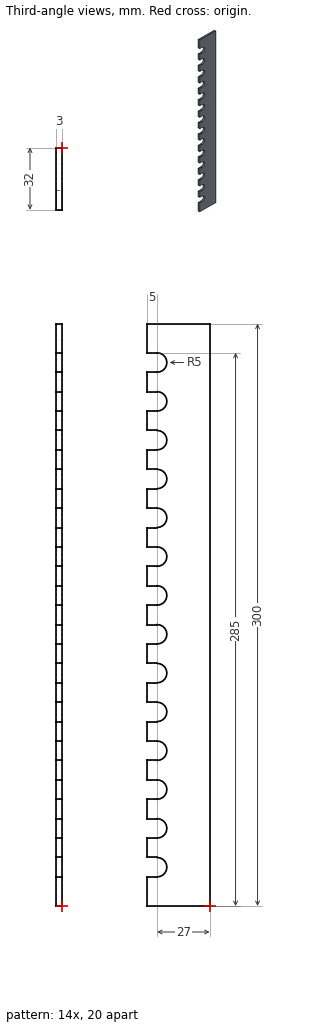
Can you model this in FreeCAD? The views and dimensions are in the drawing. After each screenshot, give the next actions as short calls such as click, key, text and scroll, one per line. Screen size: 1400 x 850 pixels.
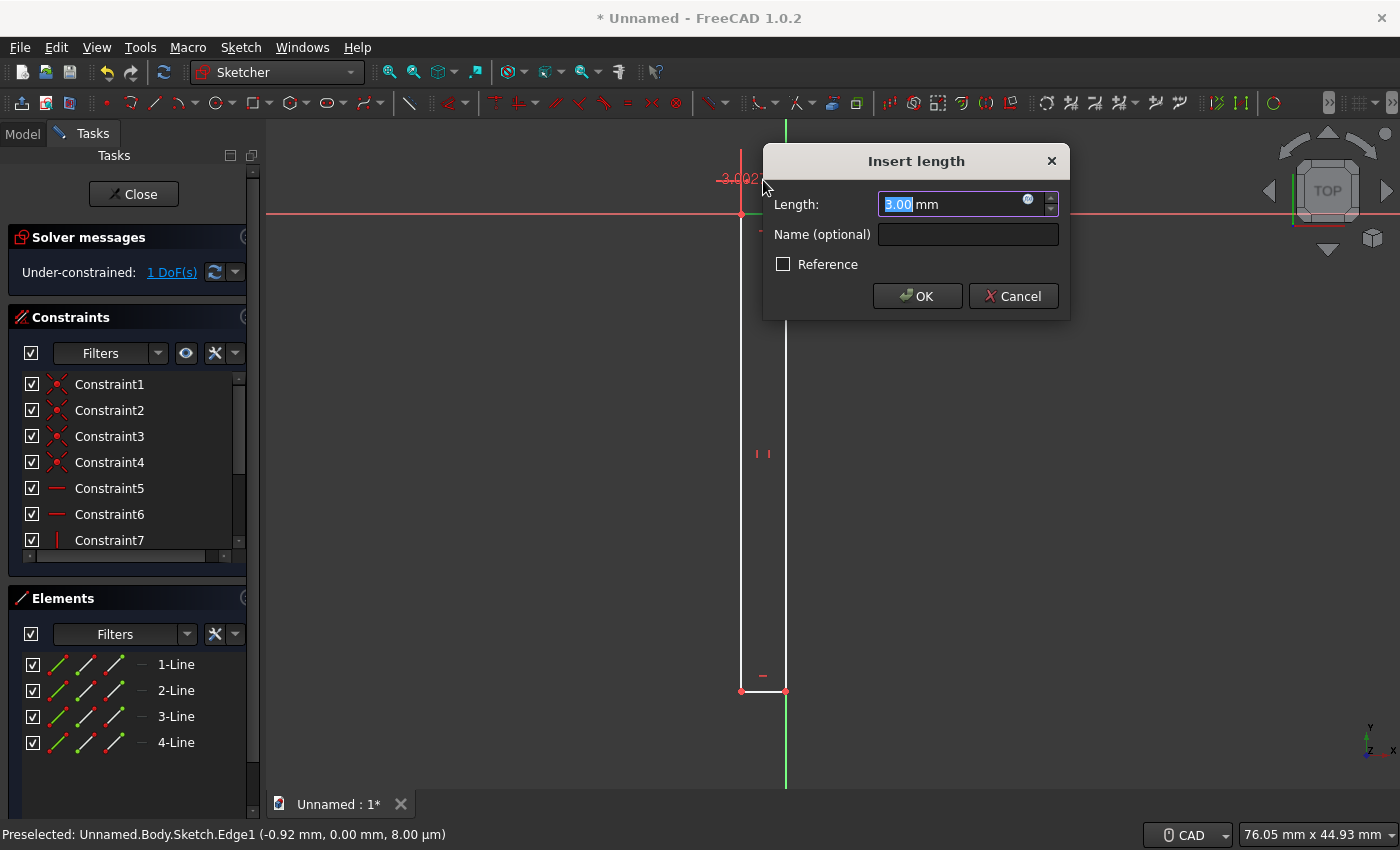
text(3)
key(Return)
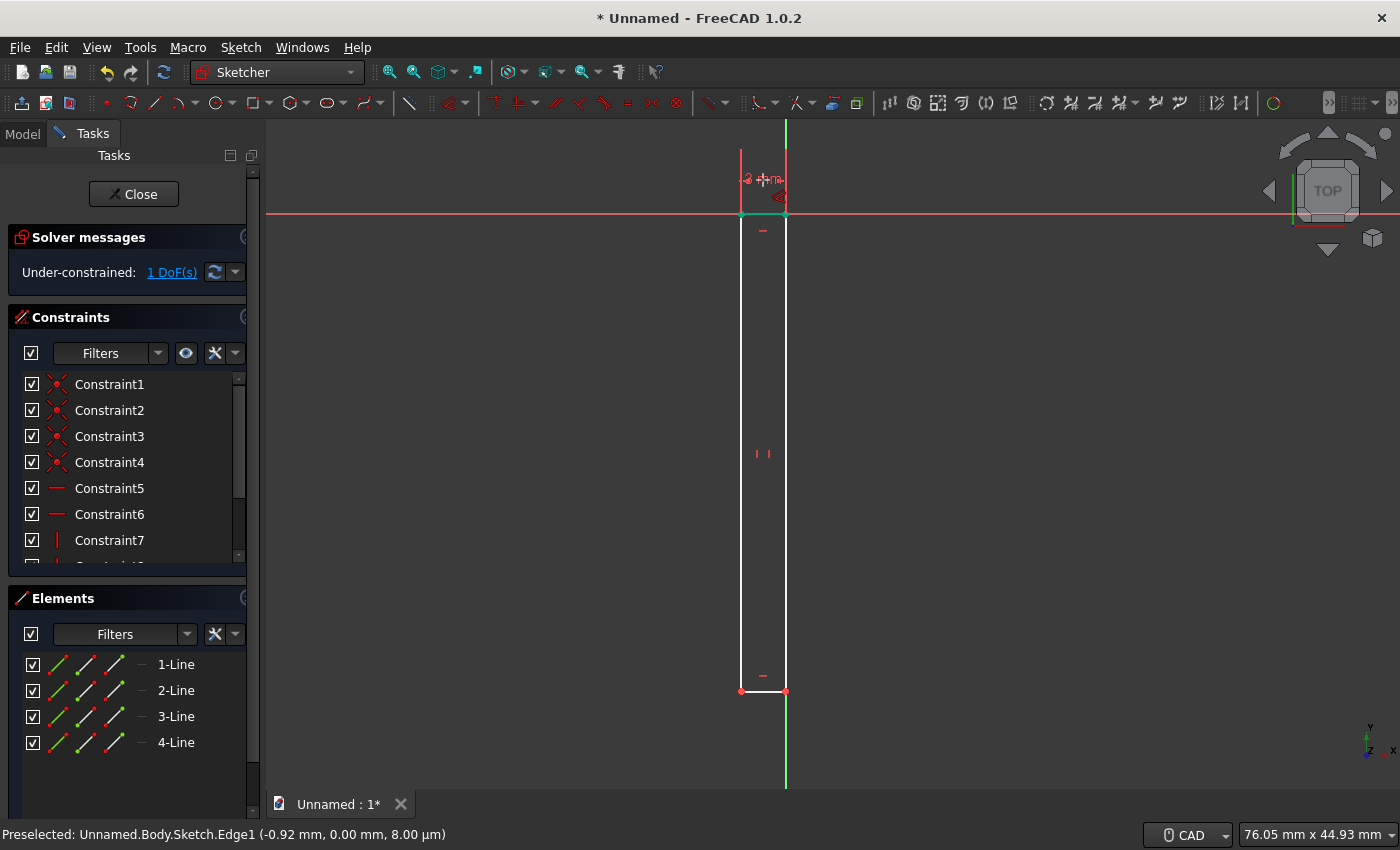
click(741, 357)
click(707, 453)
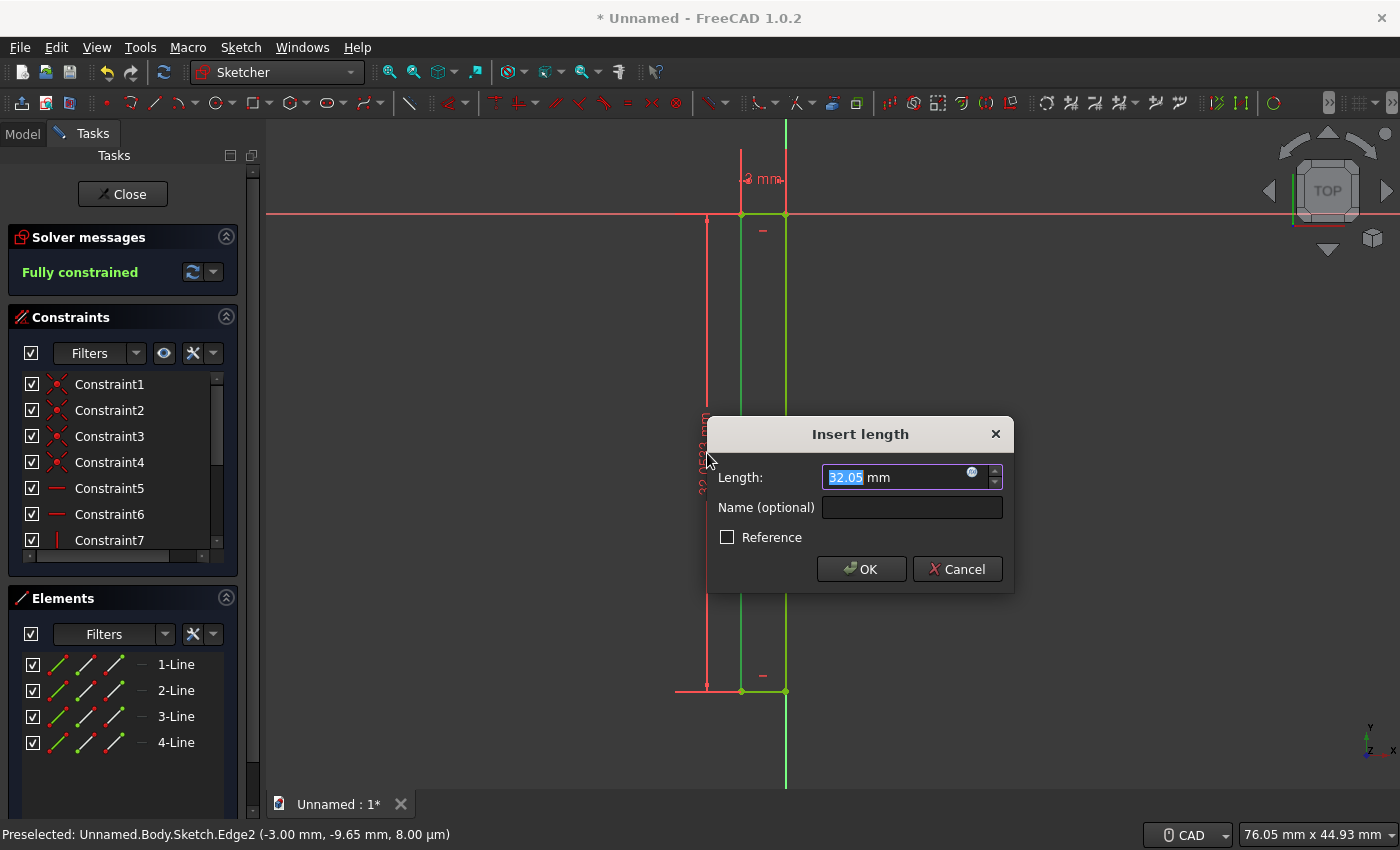
text(32)
key(Return)
key(Escape)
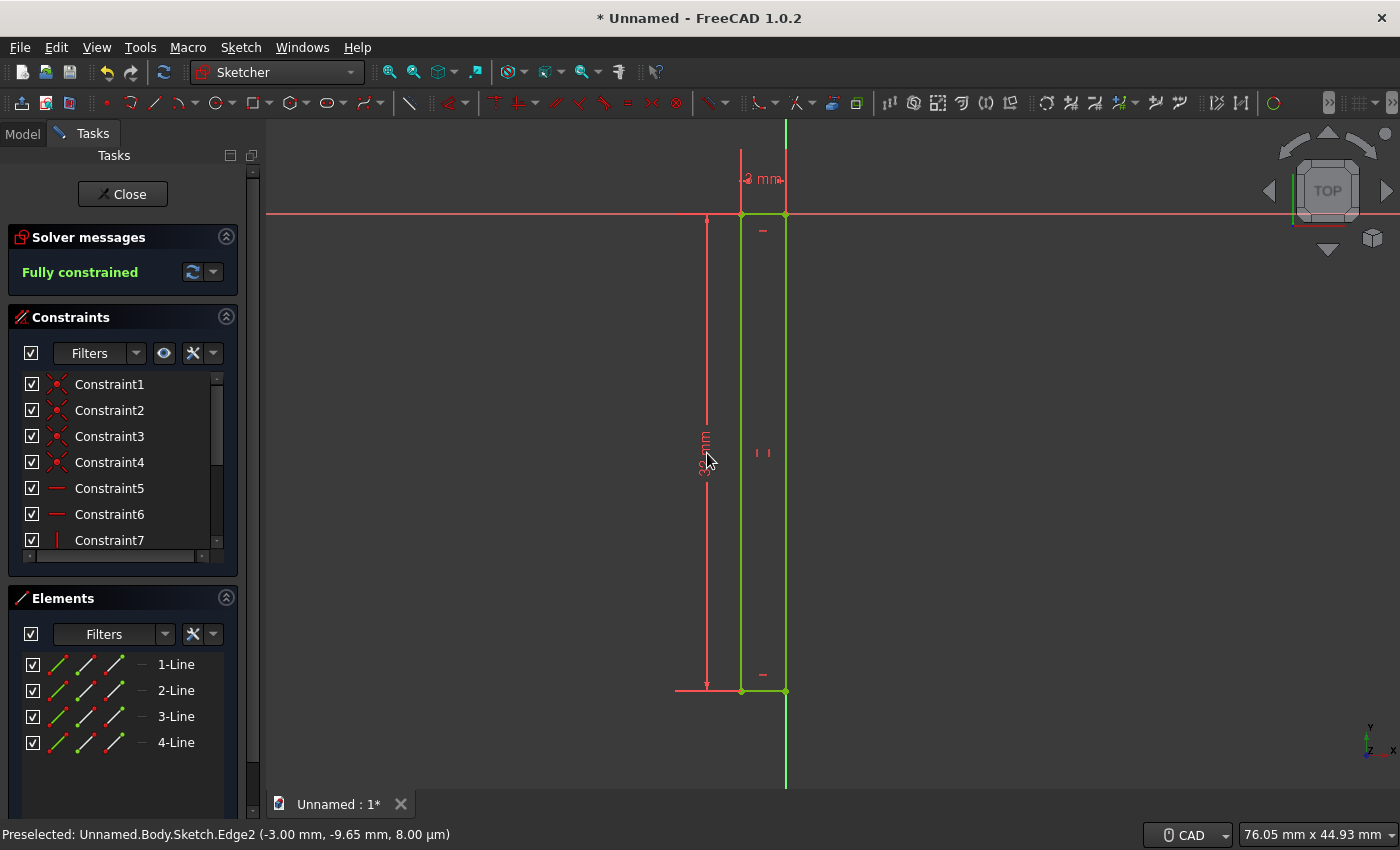
click(123, 194)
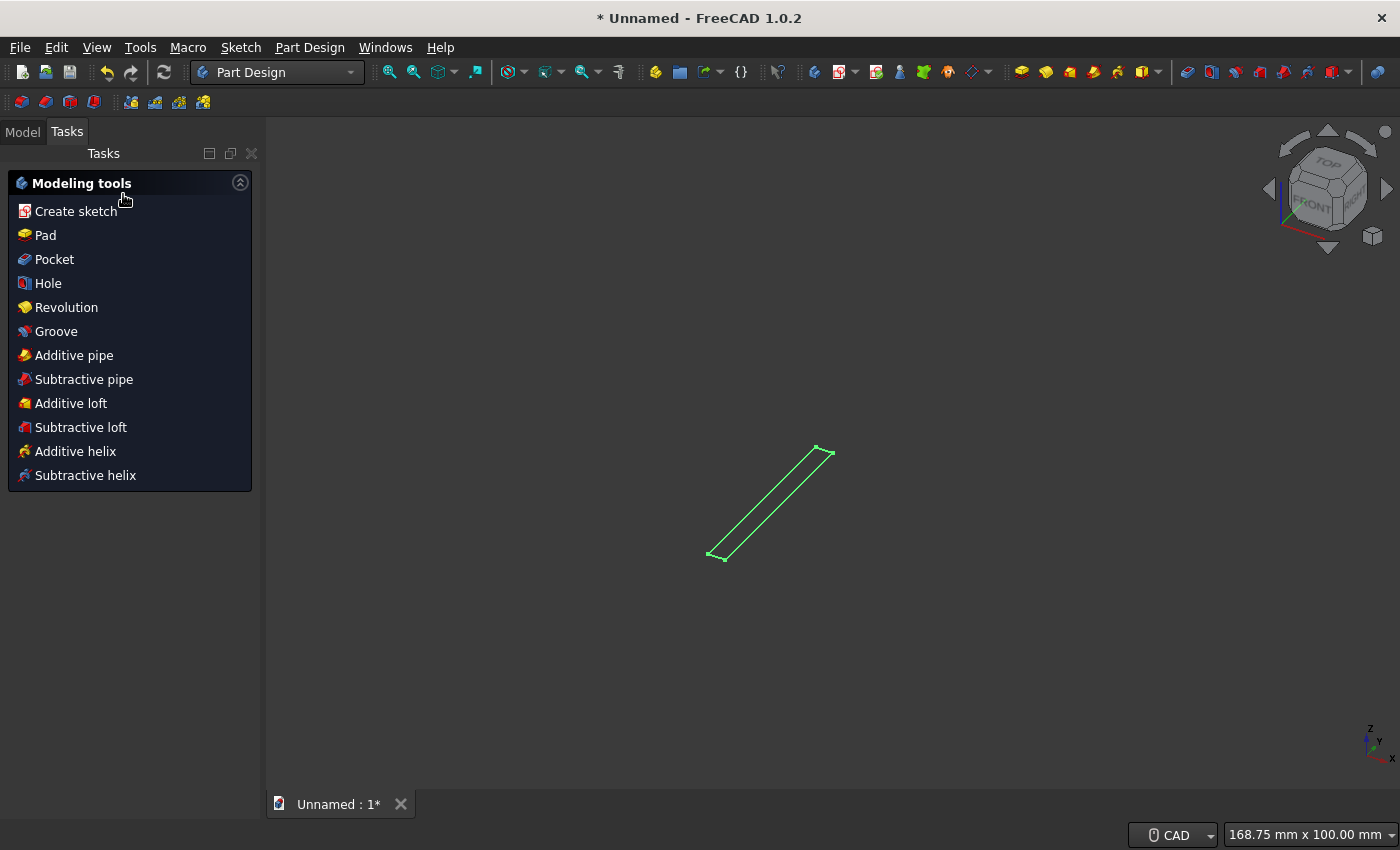
click(1022, 72)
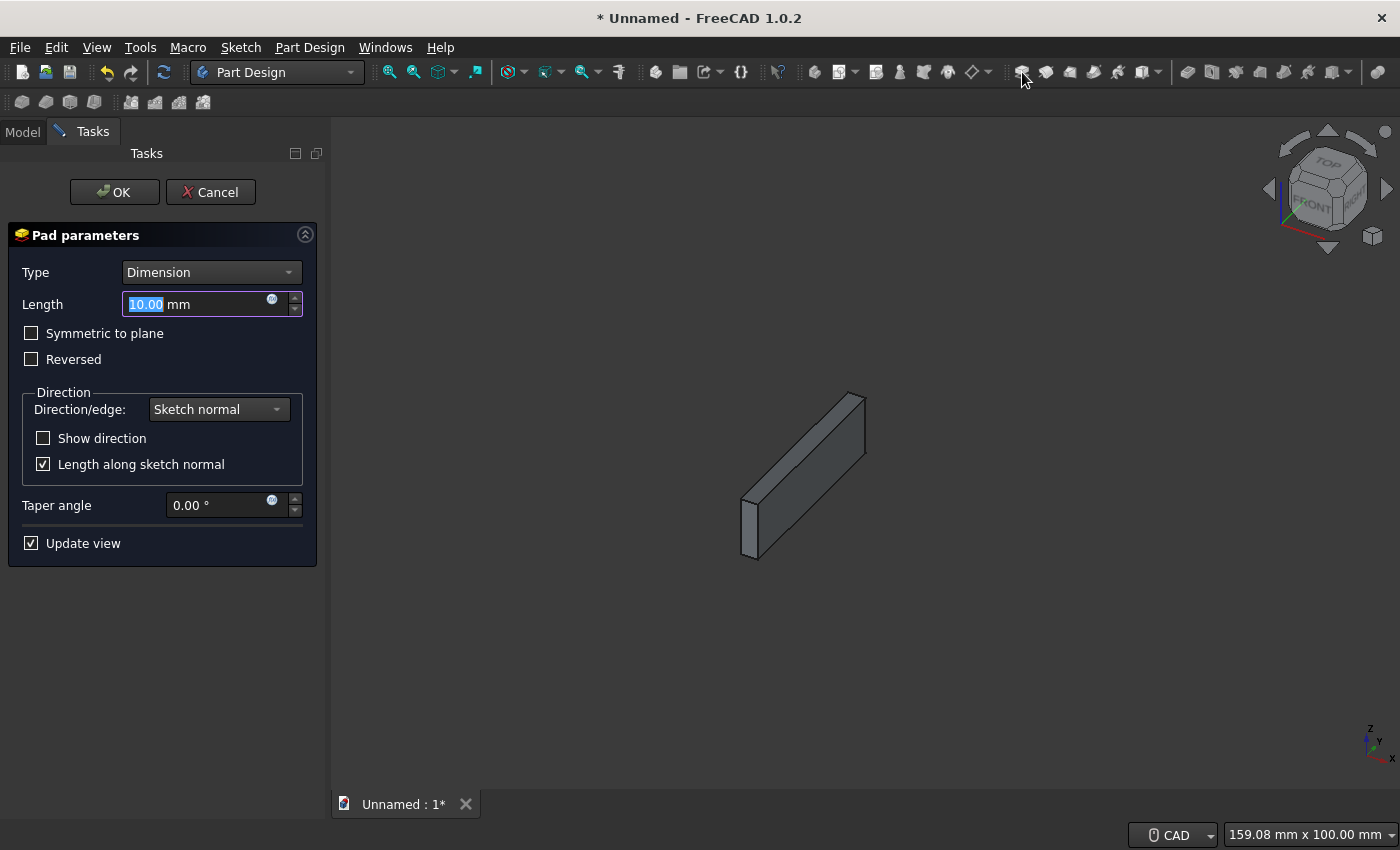
text(300)
key(Tab)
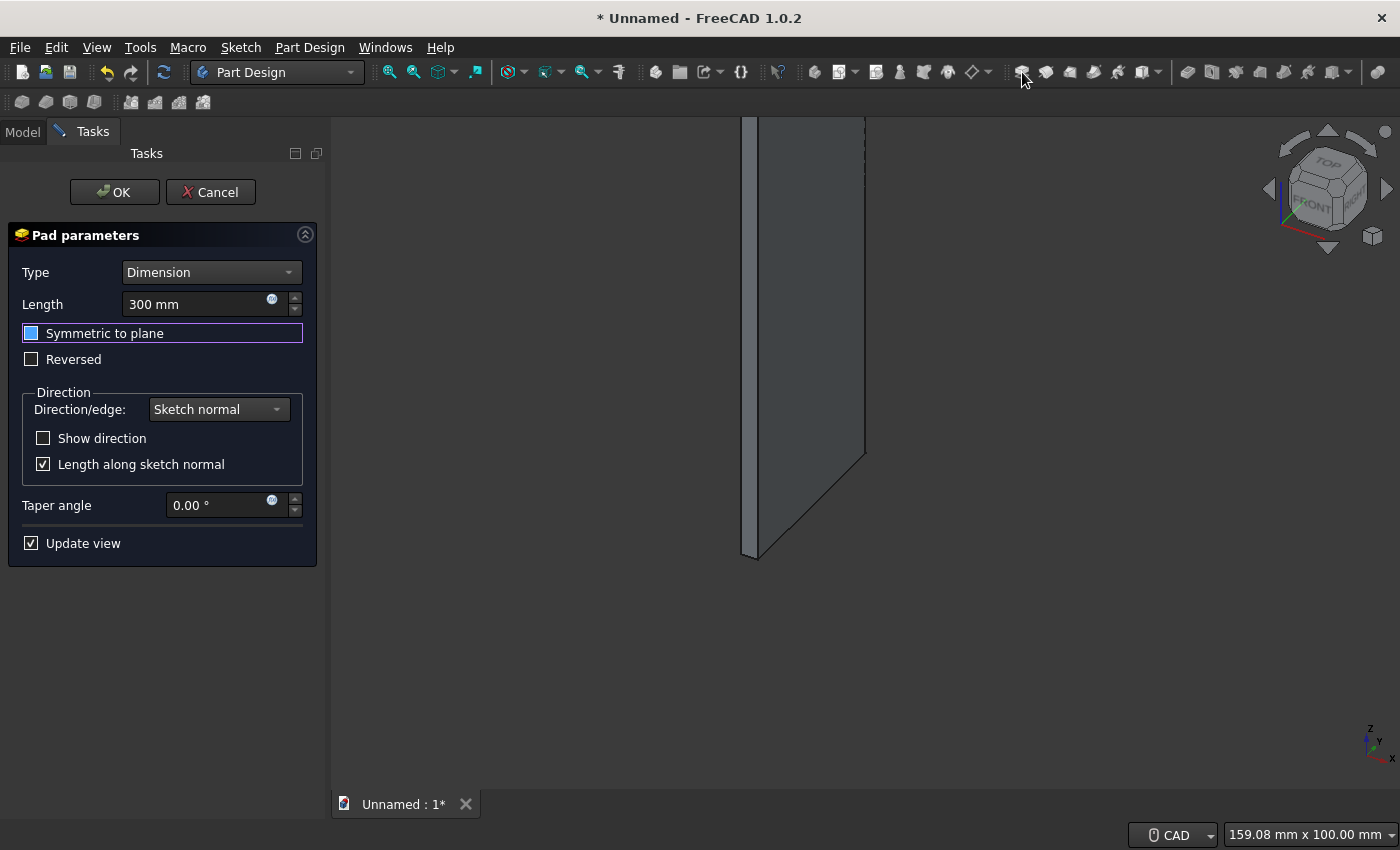
click(115, 192)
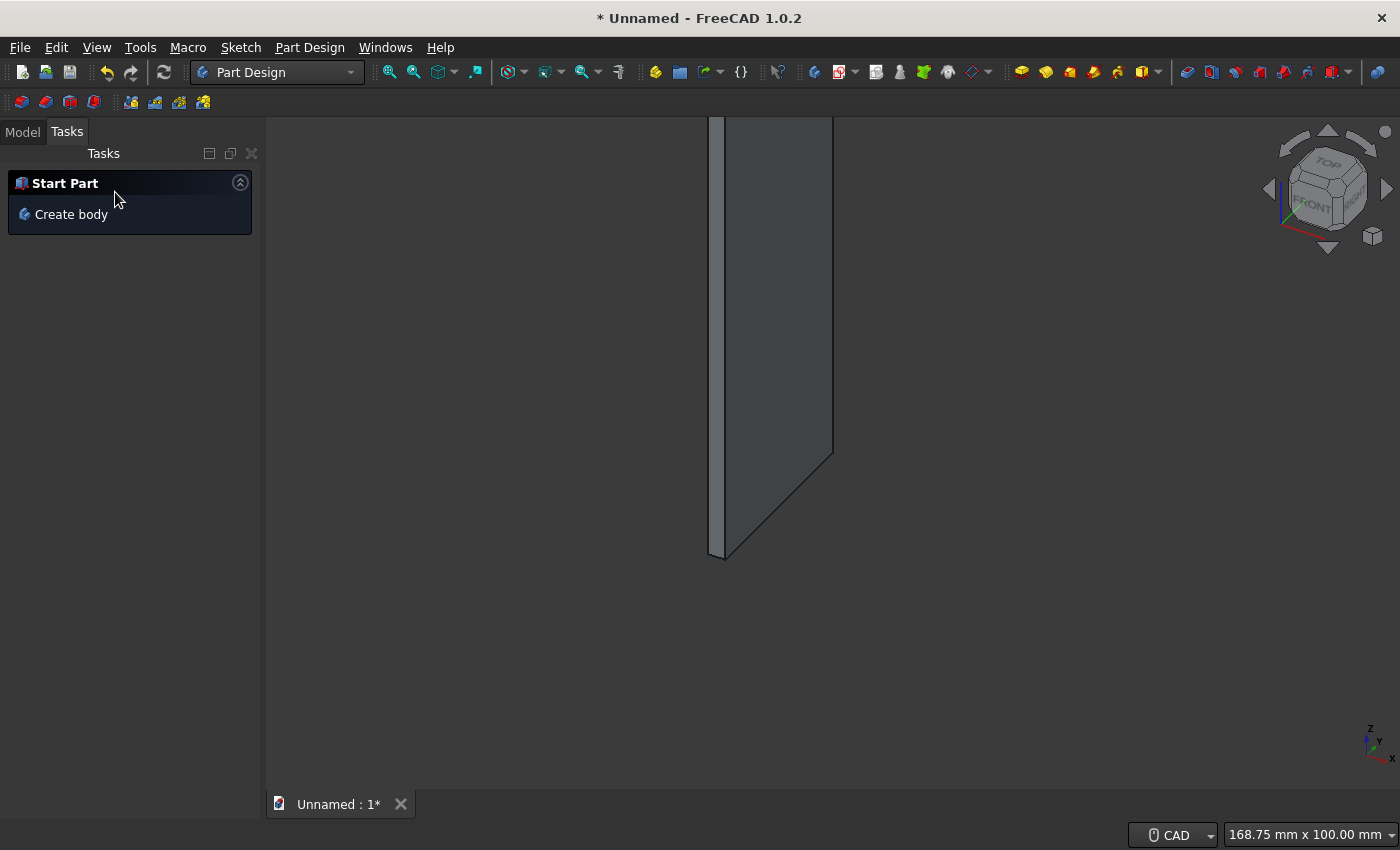
key(v)
key(f)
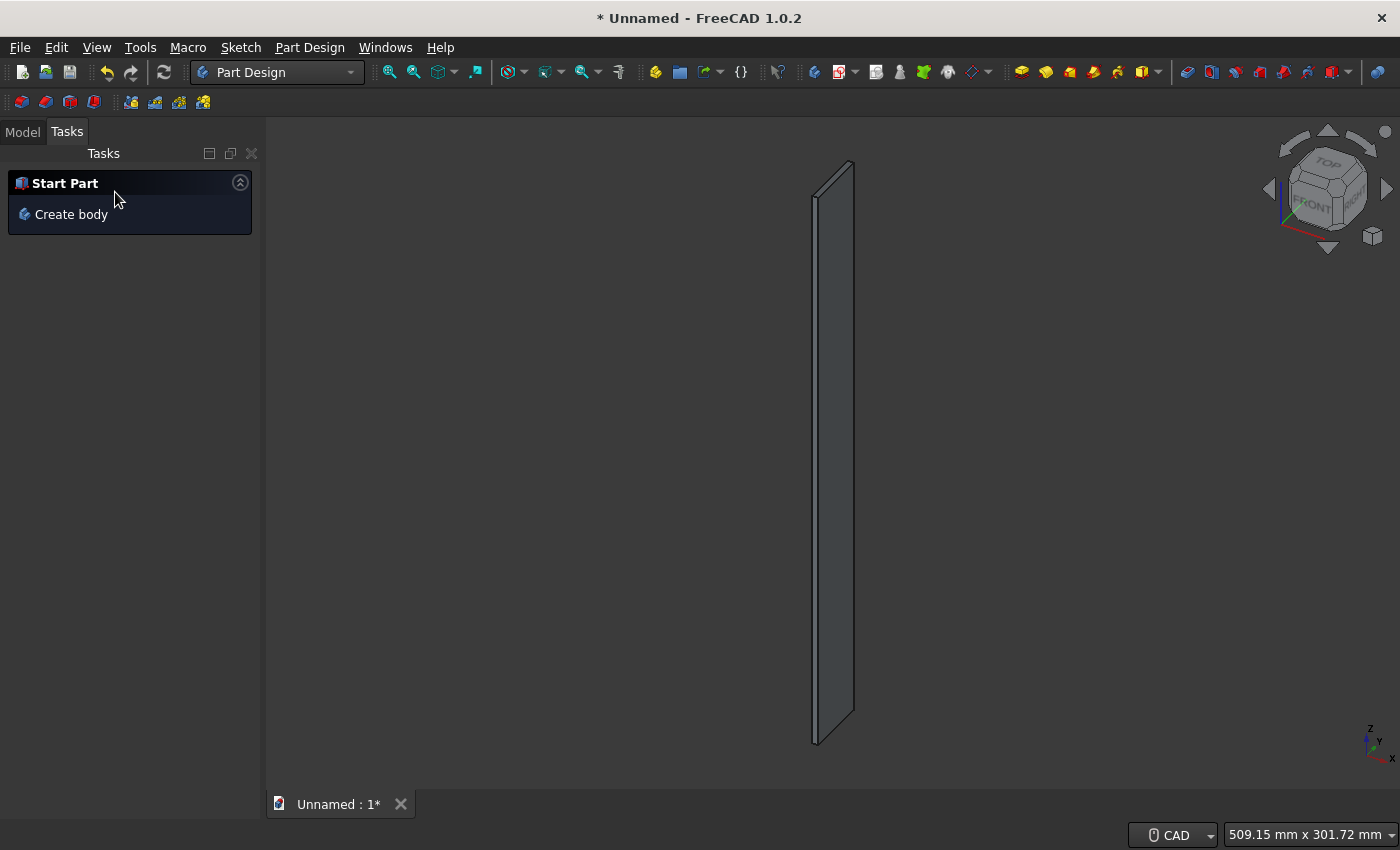
click(836, 218)